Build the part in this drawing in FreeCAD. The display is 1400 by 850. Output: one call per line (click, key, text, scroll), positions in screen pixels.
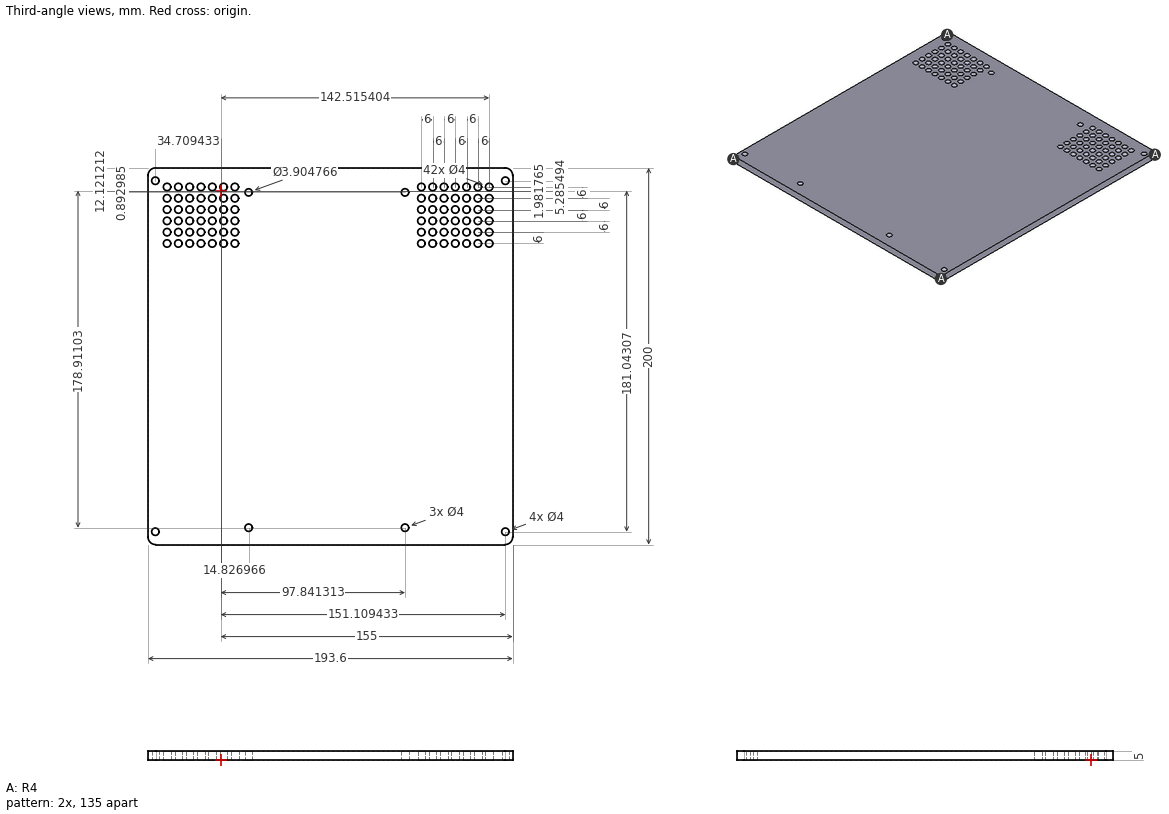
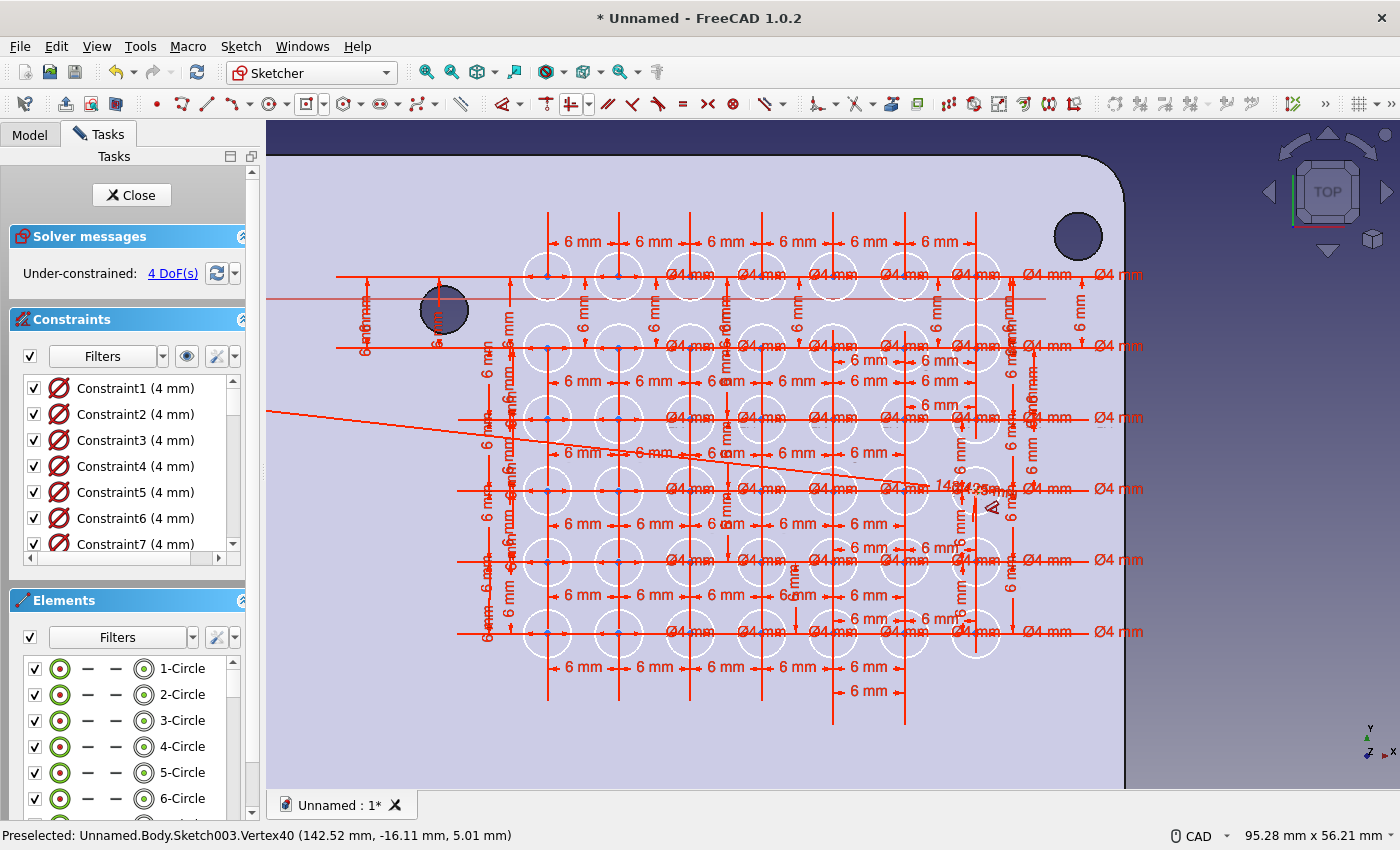
click(976, 562)
click(1034, 527)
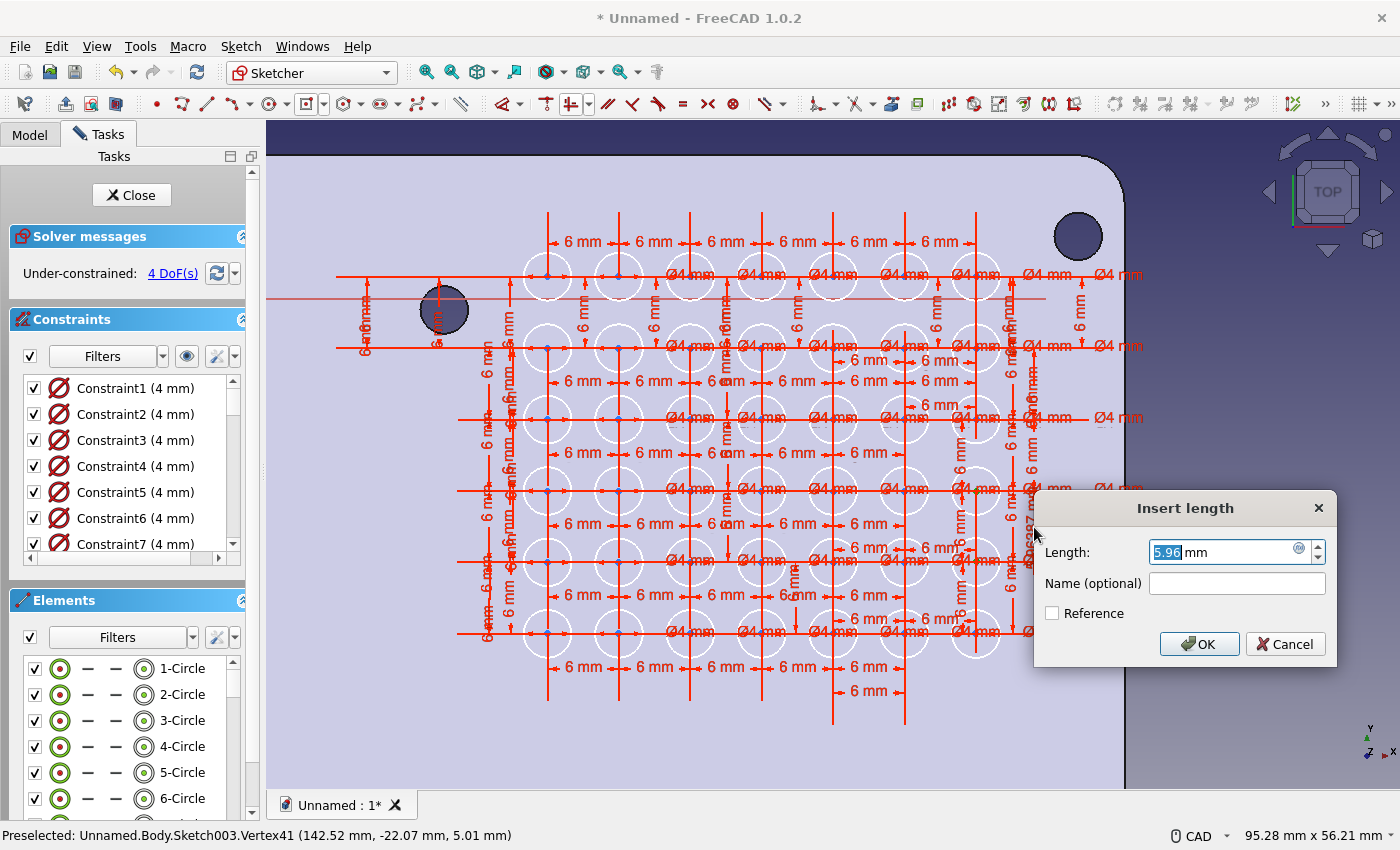
text(6)
key(Return)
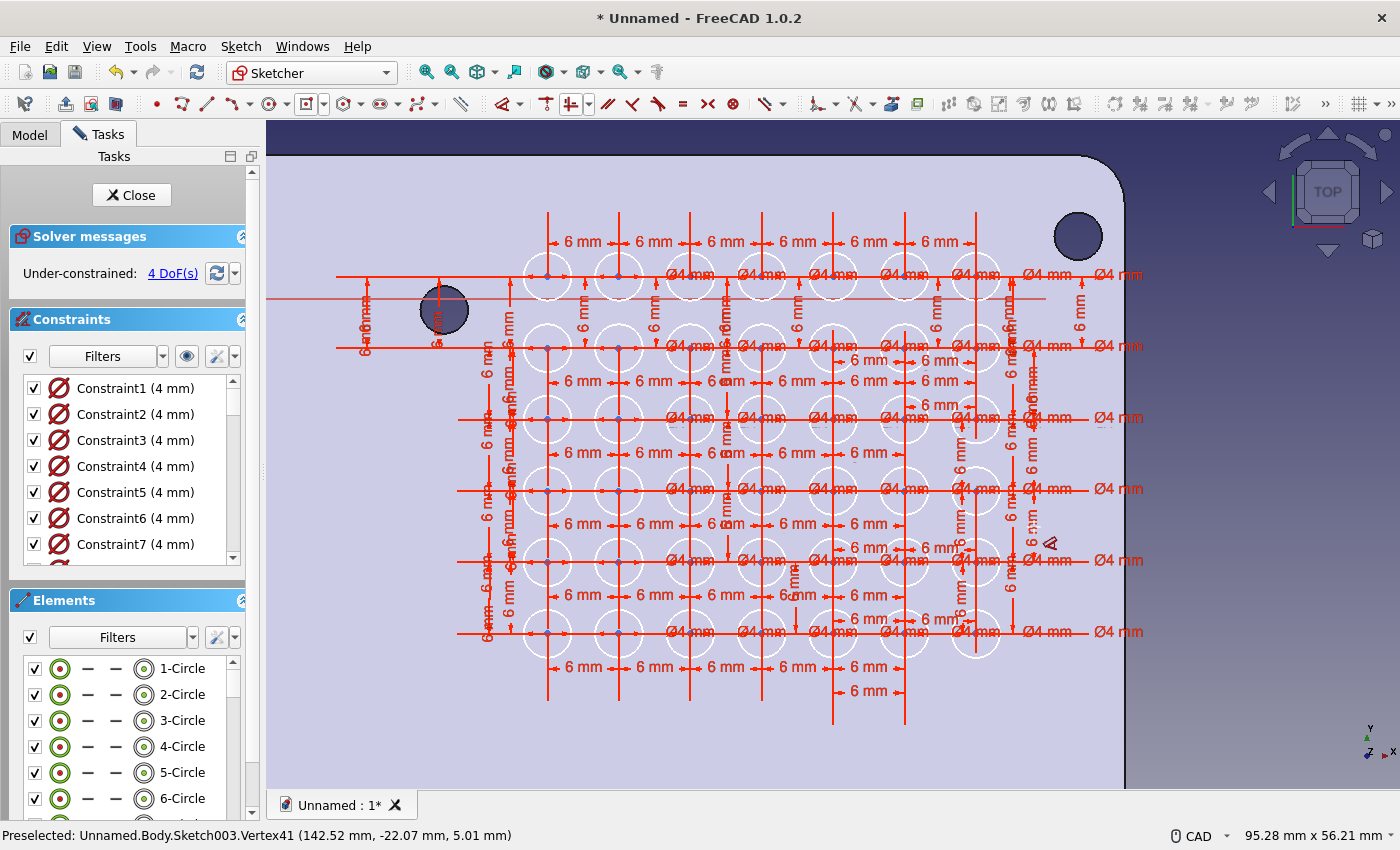
click(905, 634)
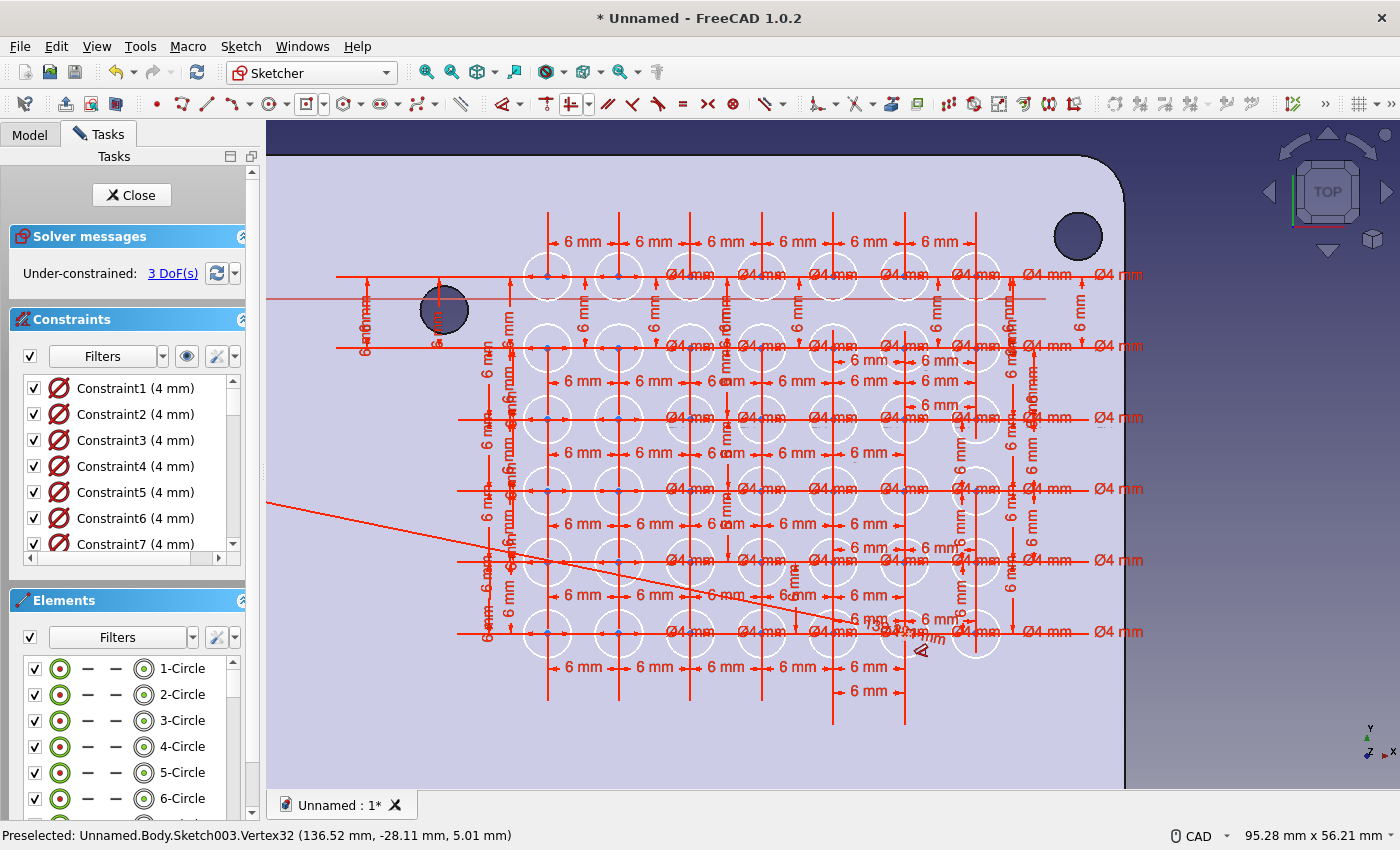
click(976, 634)
click(940, 668)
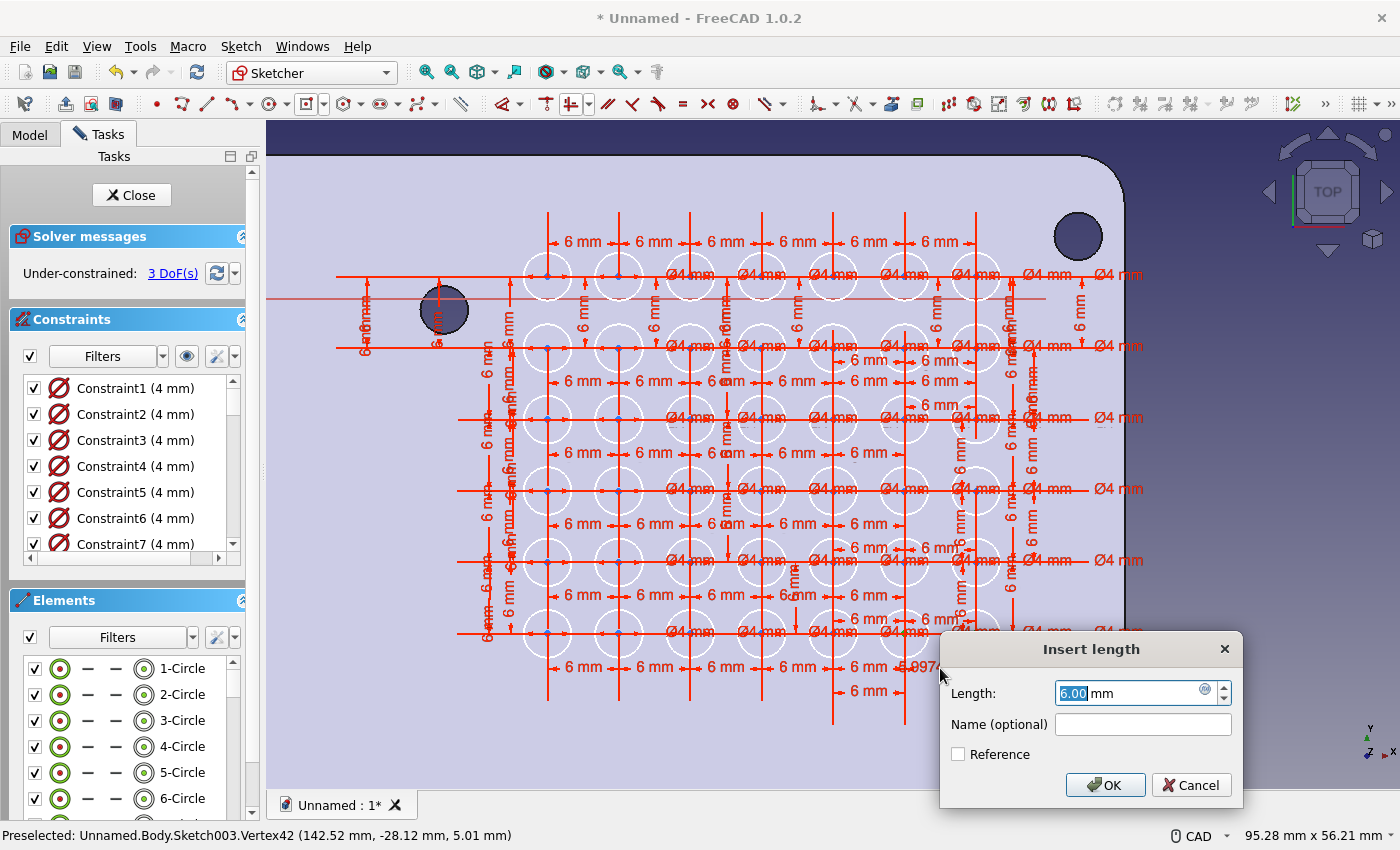
text(6)
key(Return)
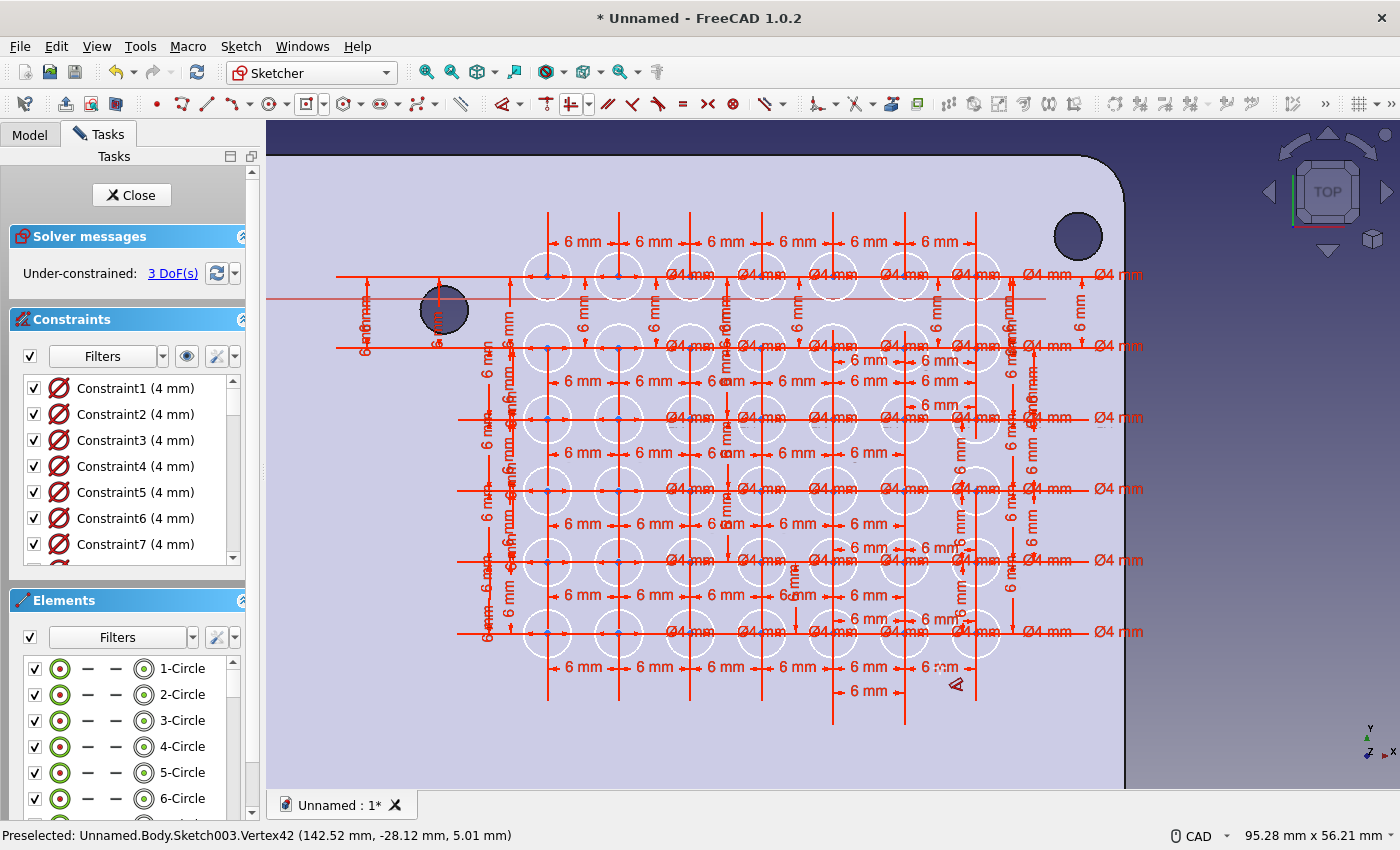
click(976, 562)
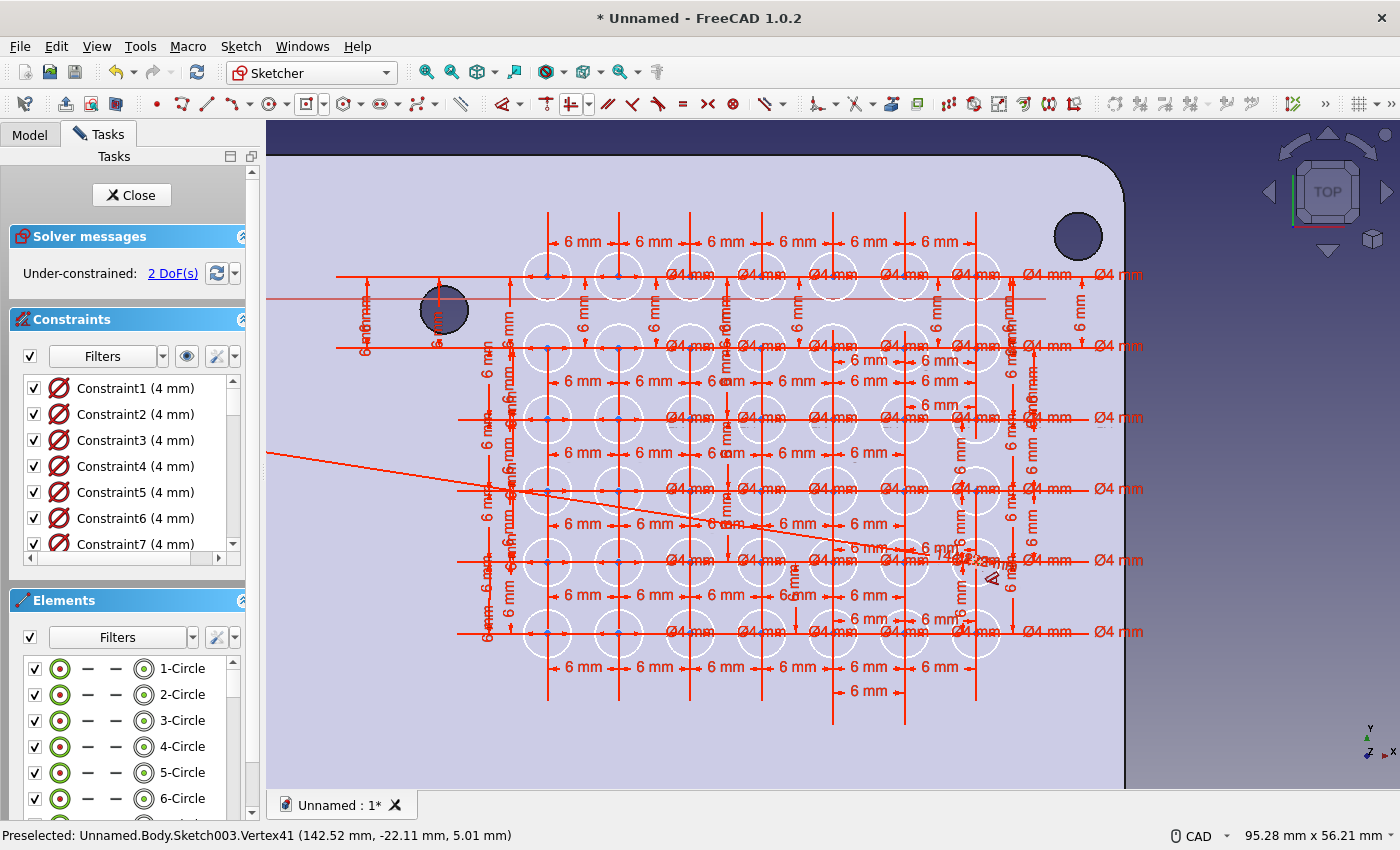
click(976, 634)
click(1034, 598)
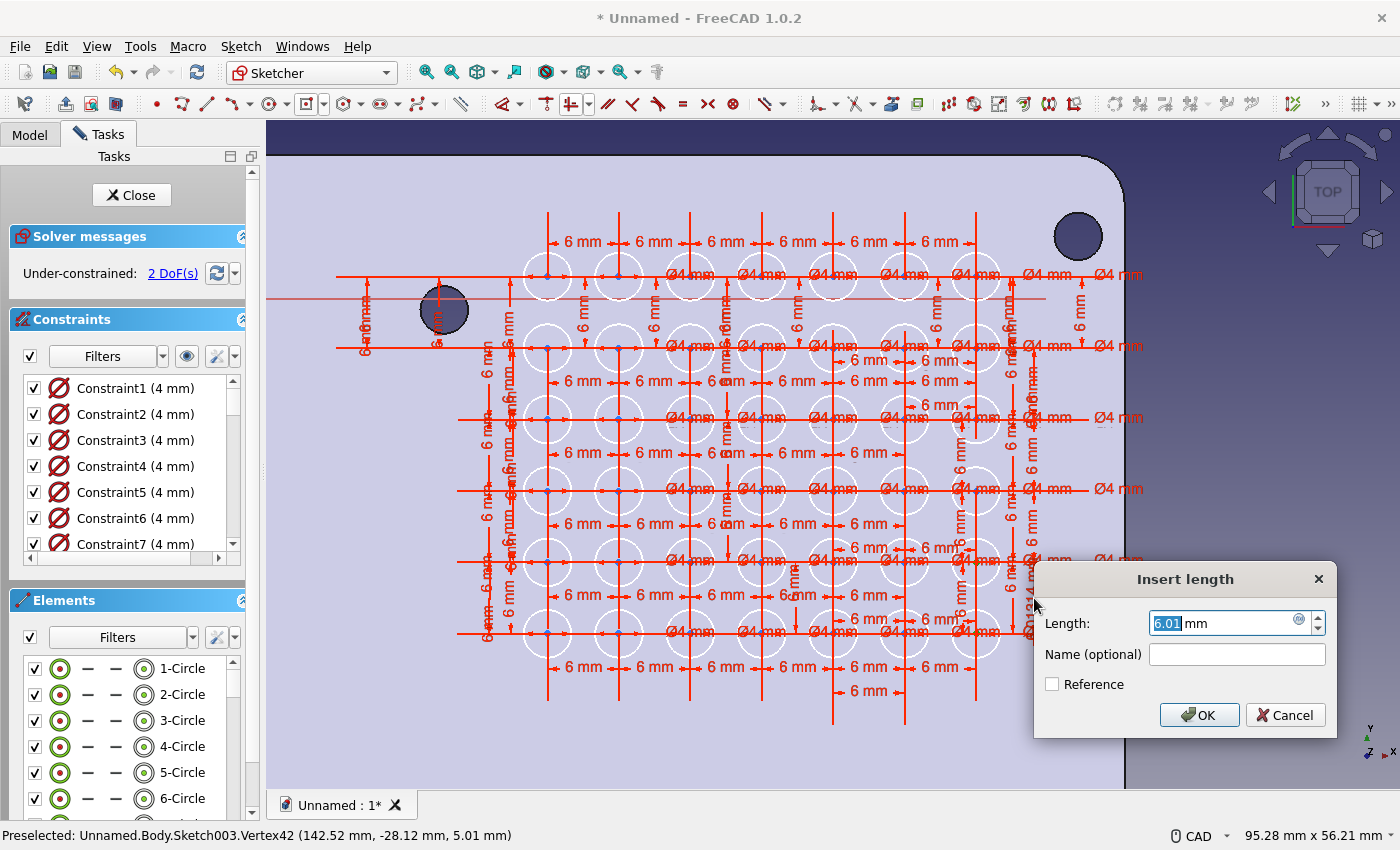
text(6)
key(Return)